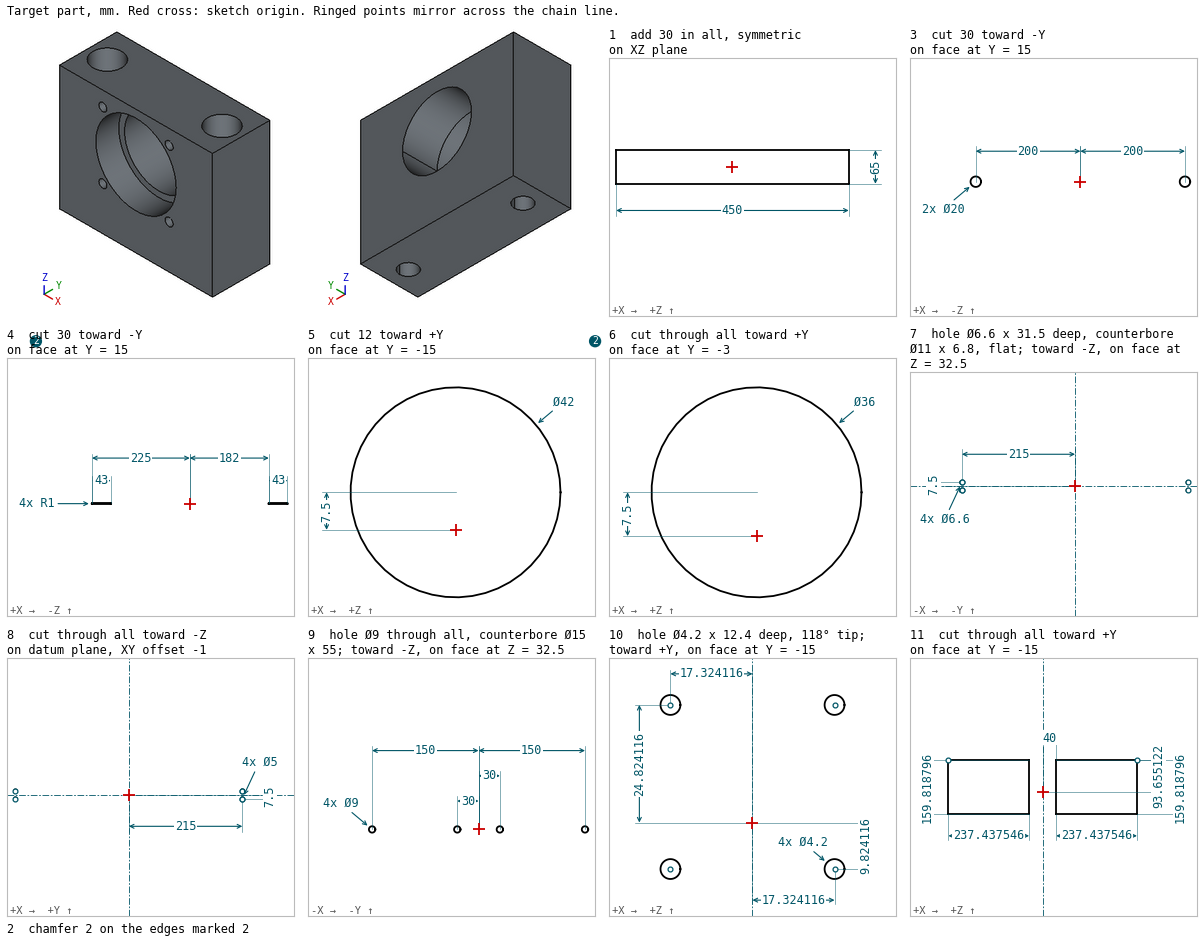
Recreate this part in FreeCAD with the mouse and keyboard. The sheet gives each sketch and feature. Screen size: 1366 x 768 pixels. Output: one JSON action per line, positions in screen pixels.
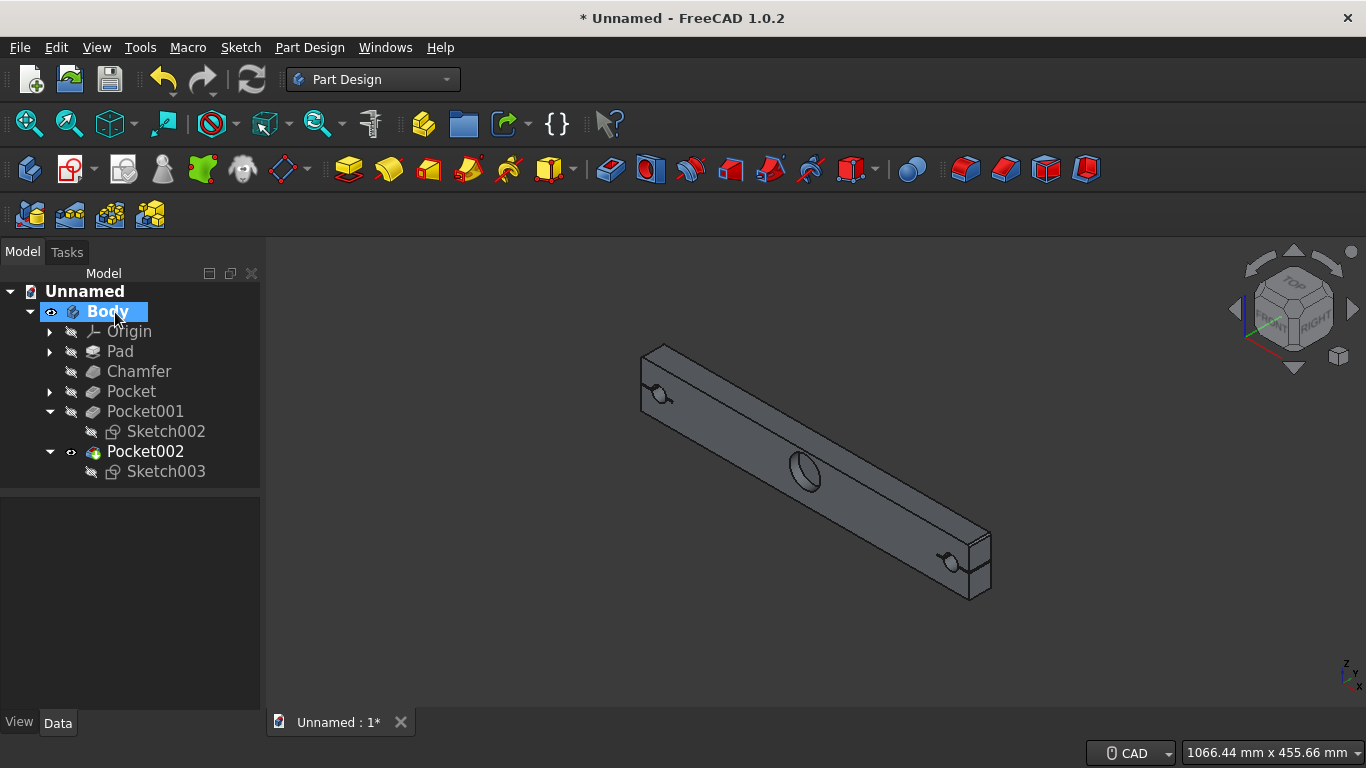
{"action": "key", "text": "1"}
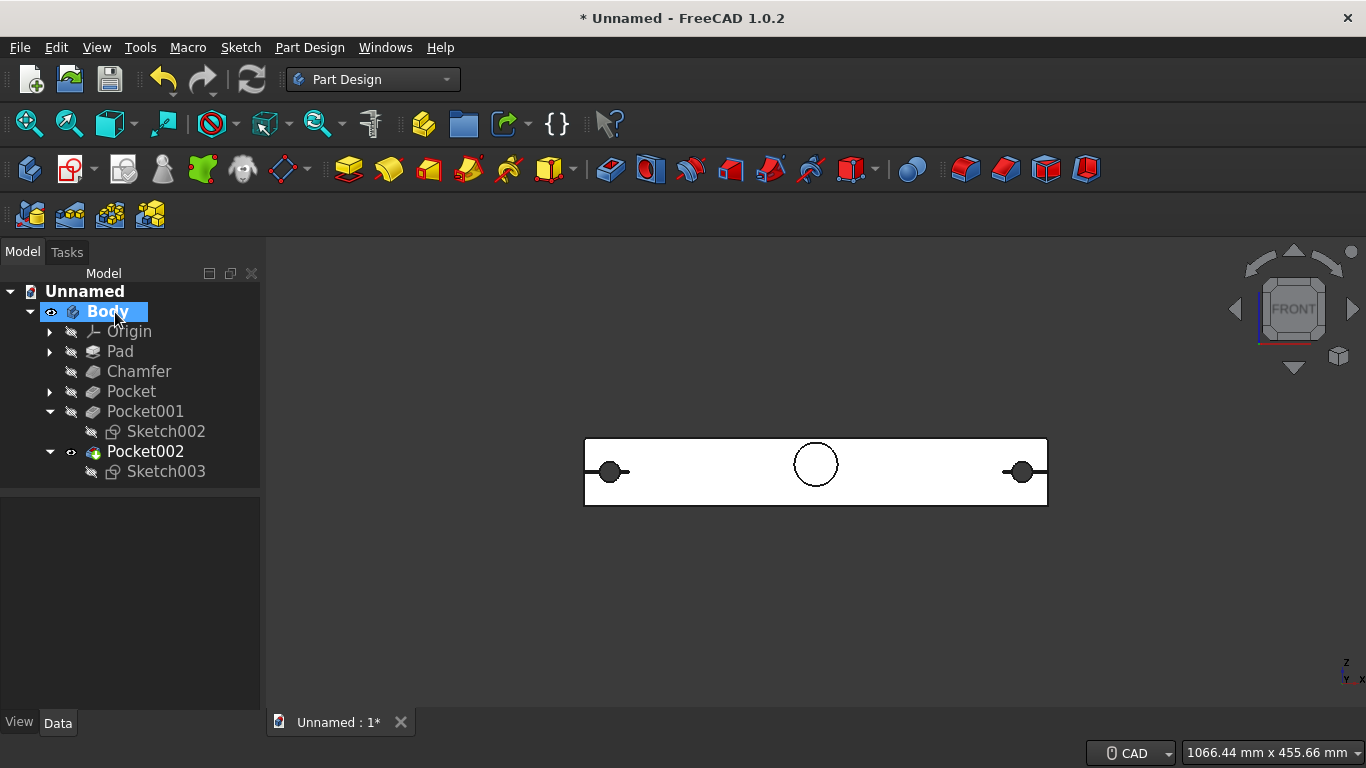
{"action": "key", "text": "v f"}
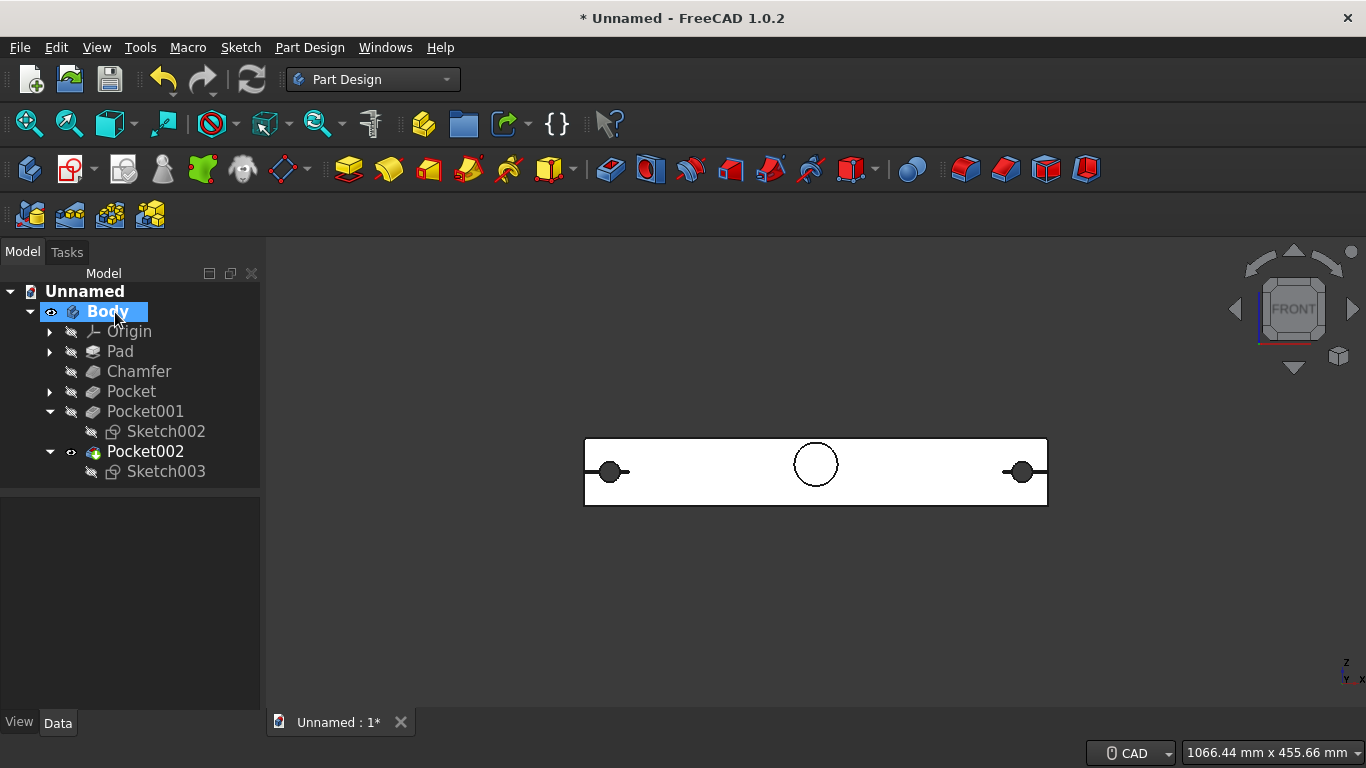
{"action": "left_click", "coordinate": [816, 463]}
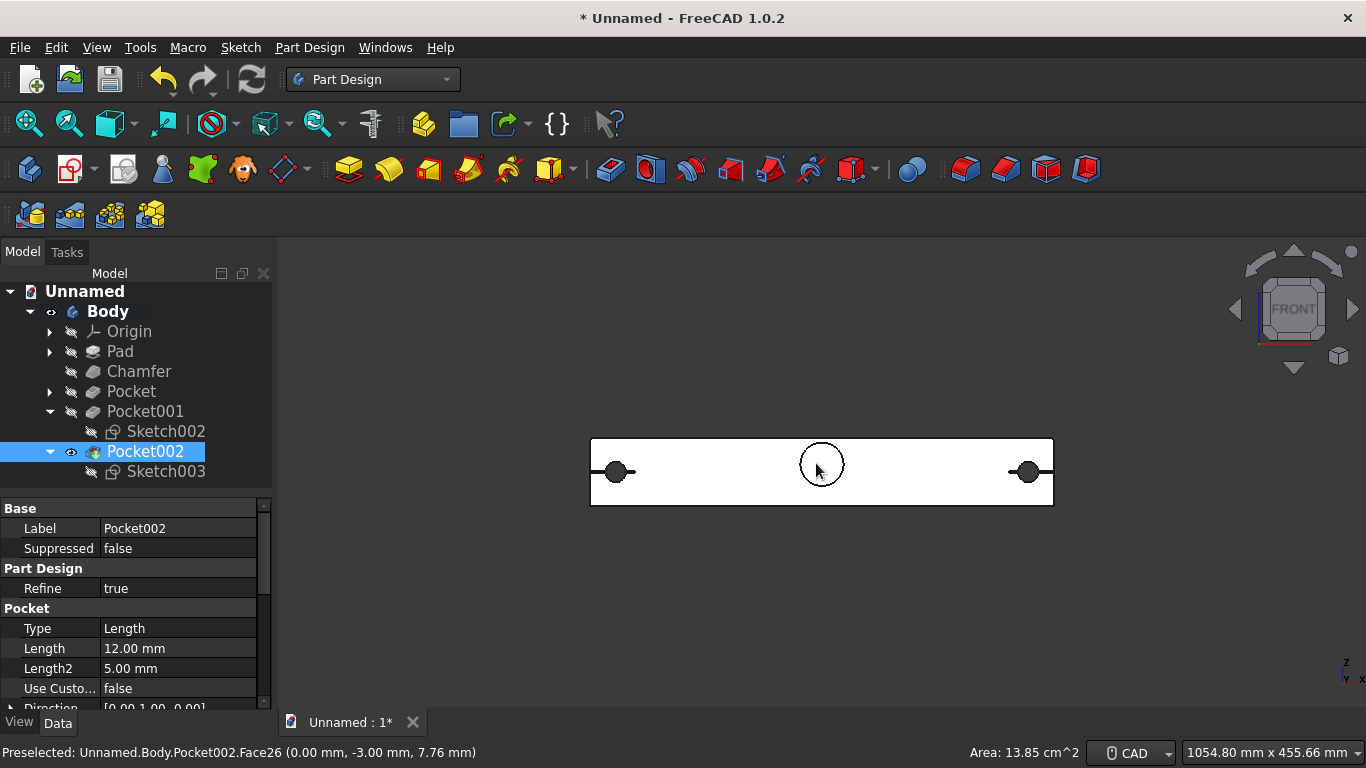
{"action": "left_click", "coordinate": [70, 170]}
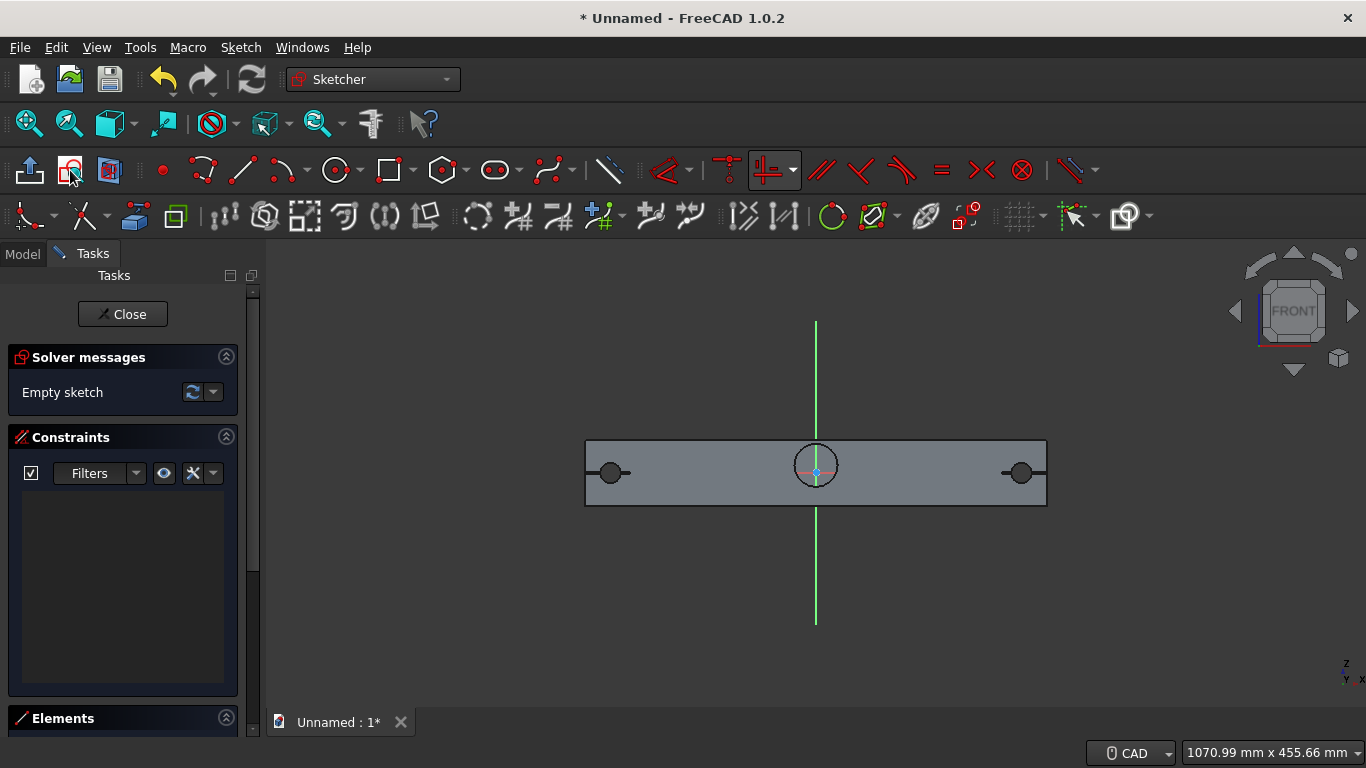
{"action": "left_click", "coordinate": [110, 170]}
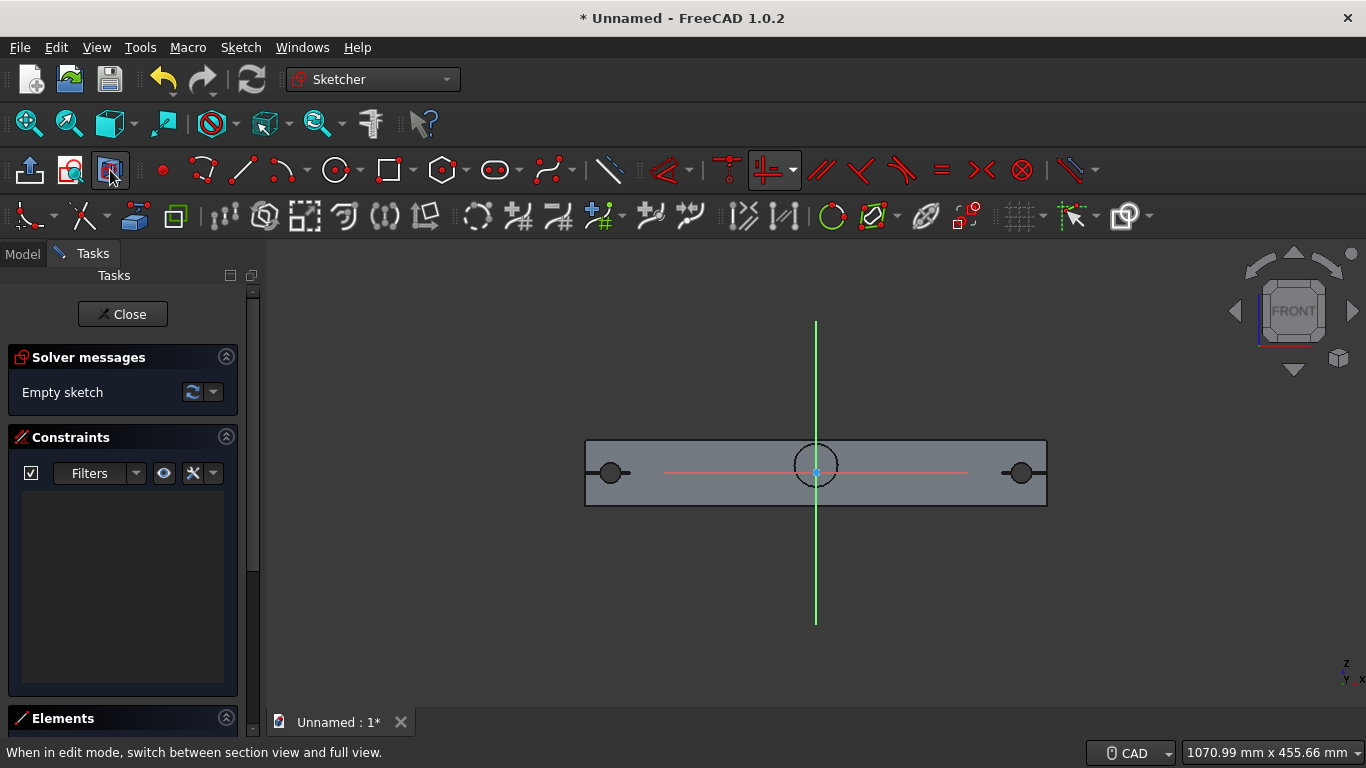
{"action": "scroll", "coordinate": [827, 464], "scroll_direction": "up", "scroll_amount": 10}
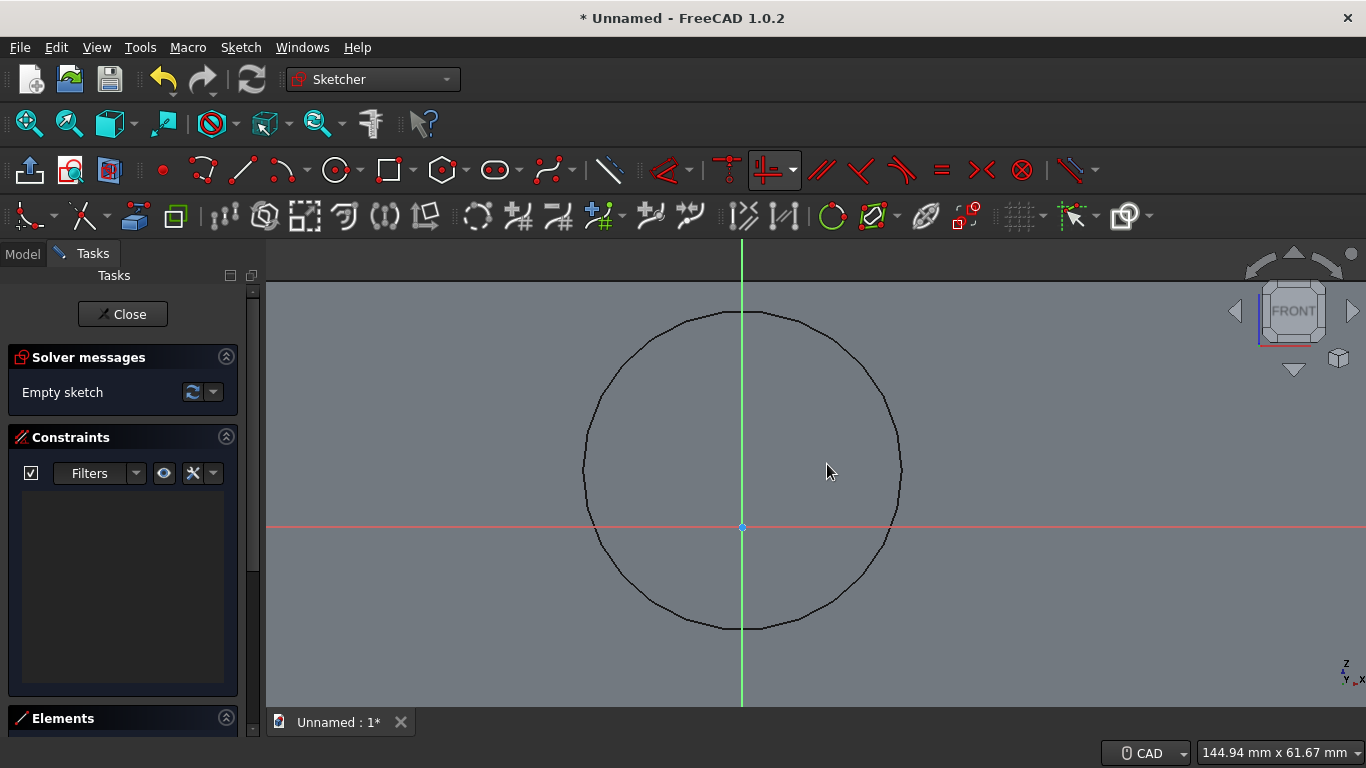
{"action": "key", "text": "g c"}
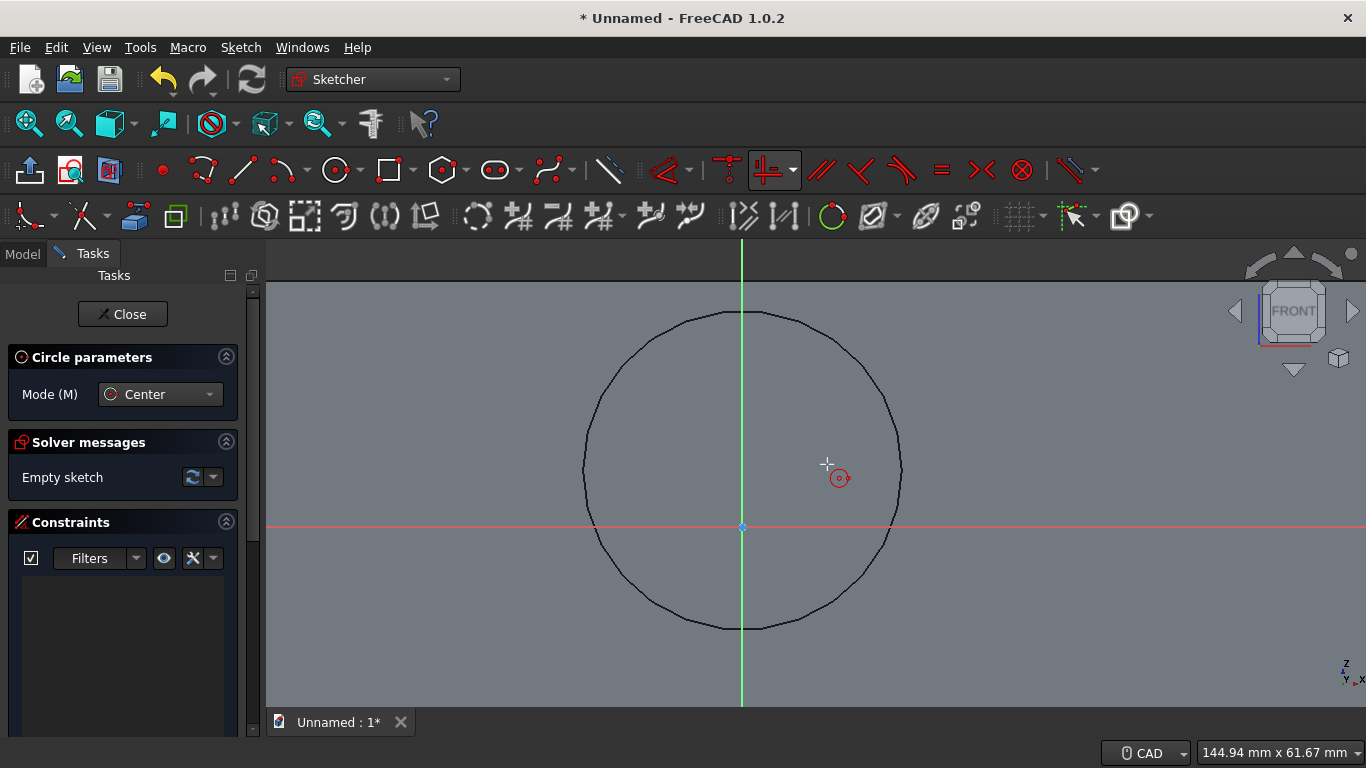
{"action": "left_click", "coordinate": [742, 471]}
{"action": "mouse_move", "coordinate": [839, 374]}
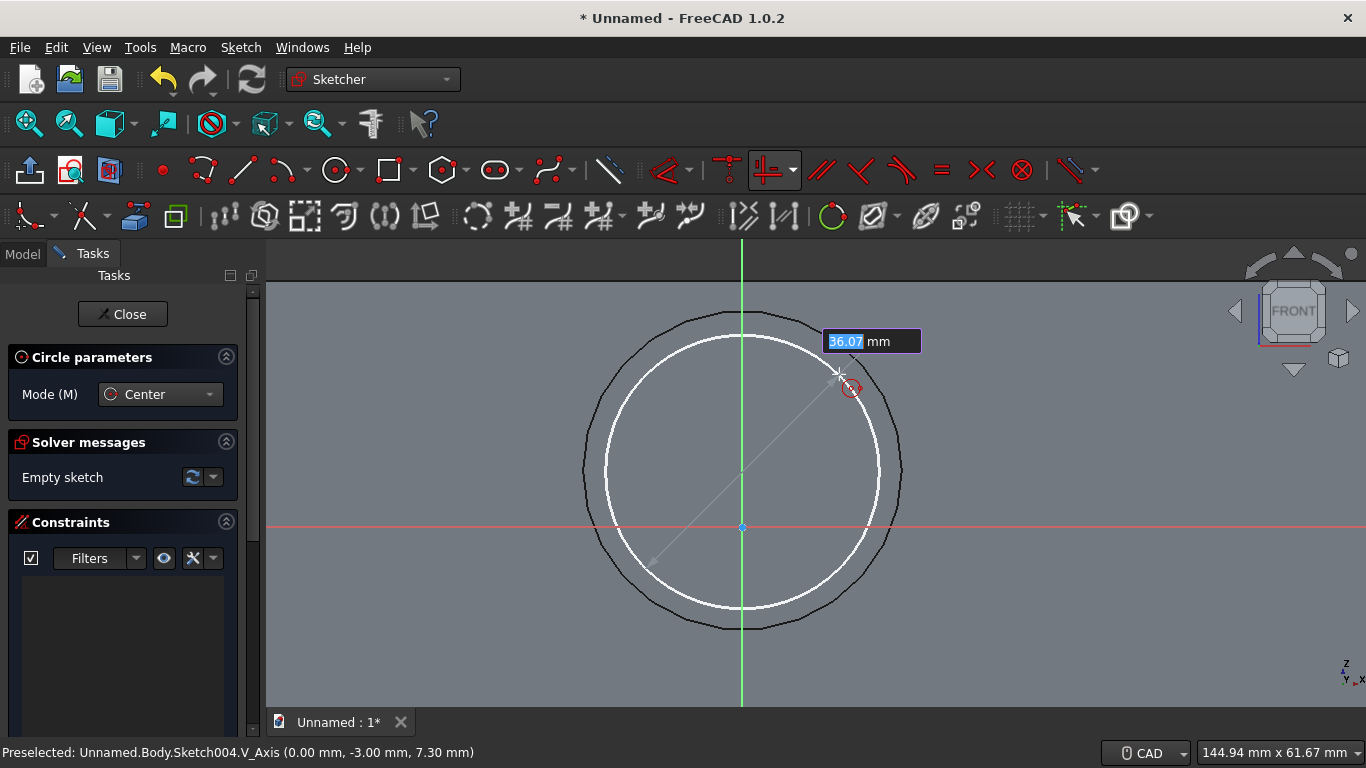
{"action": "type", "text": "36"}
{"action": "key", "text": "Return"}
{"action": "key", "text": "Escape"}